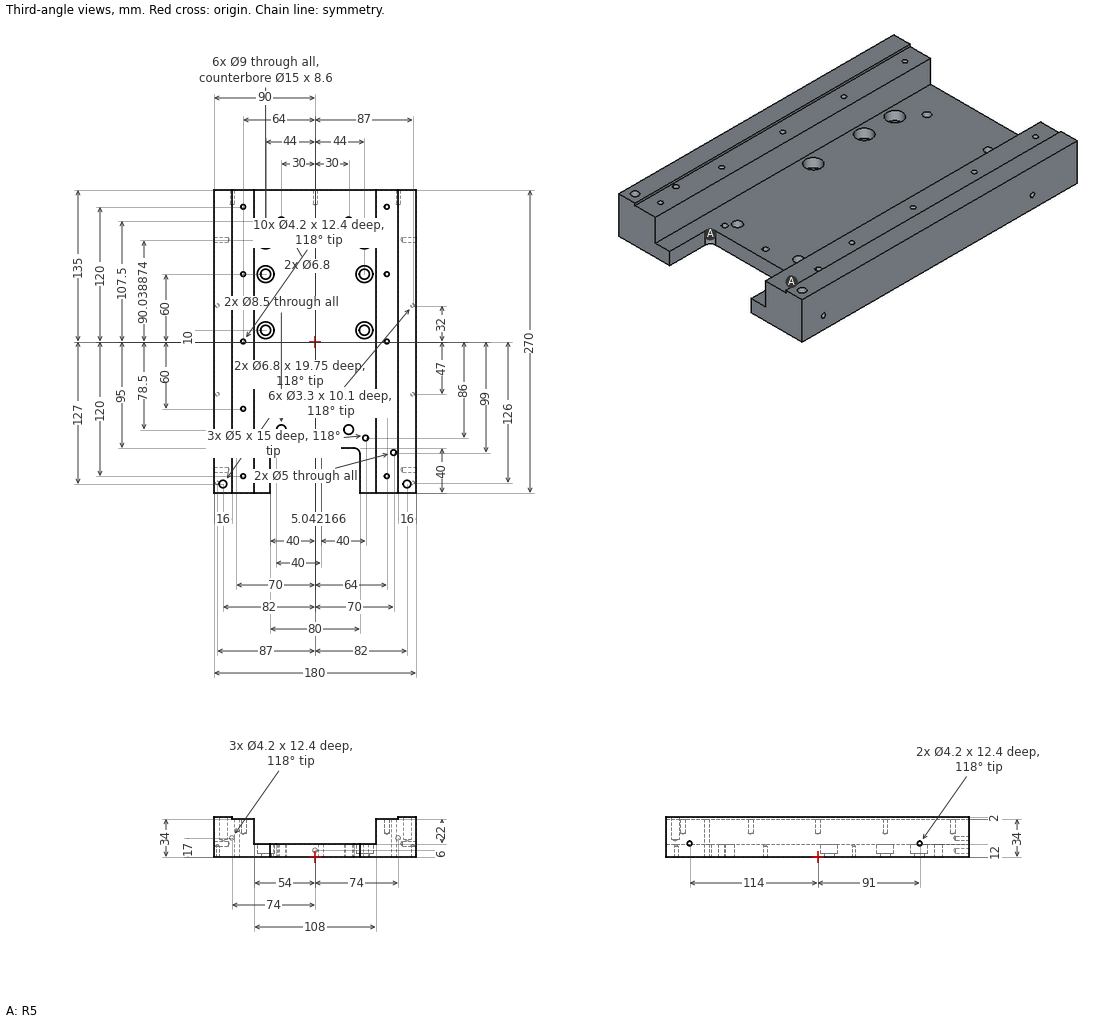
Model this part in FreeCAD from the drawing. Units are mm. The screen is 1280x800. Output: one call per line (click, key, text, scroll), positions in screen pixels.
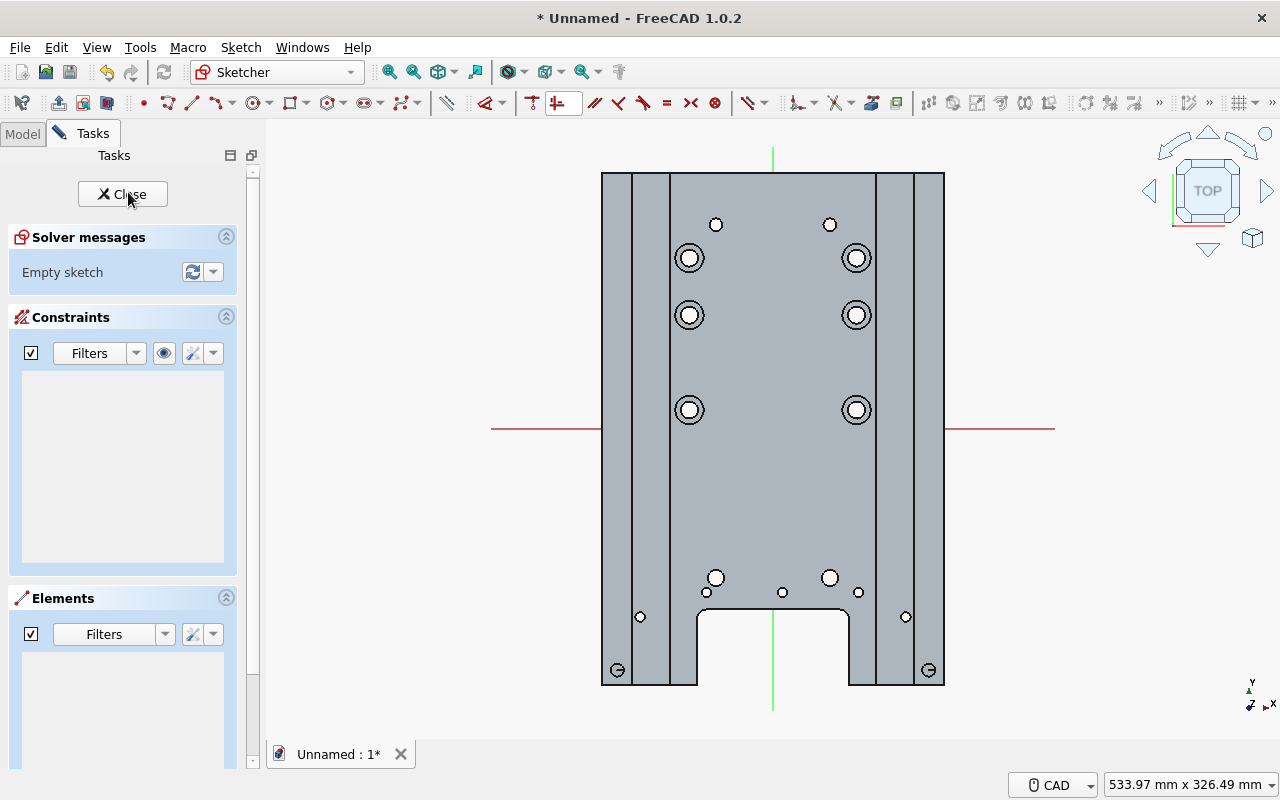
click(108, 104)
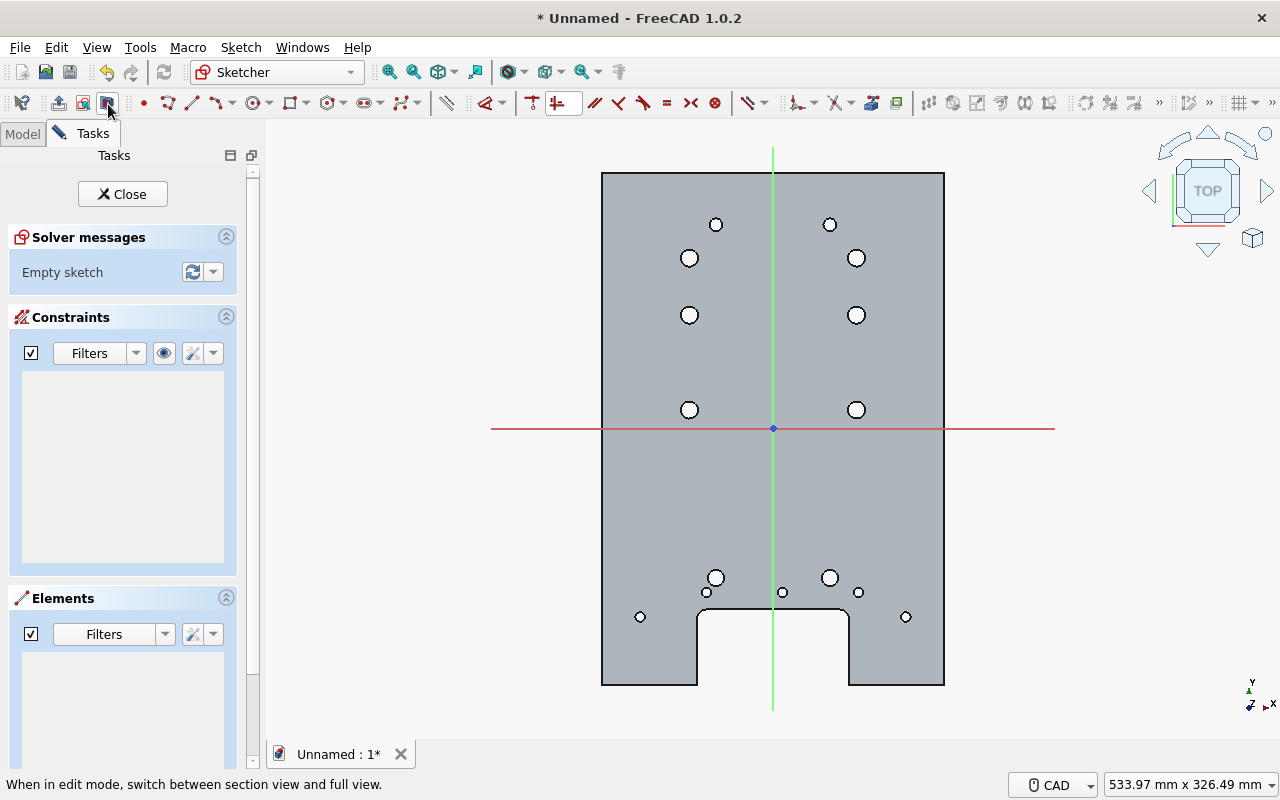
click(254, 104)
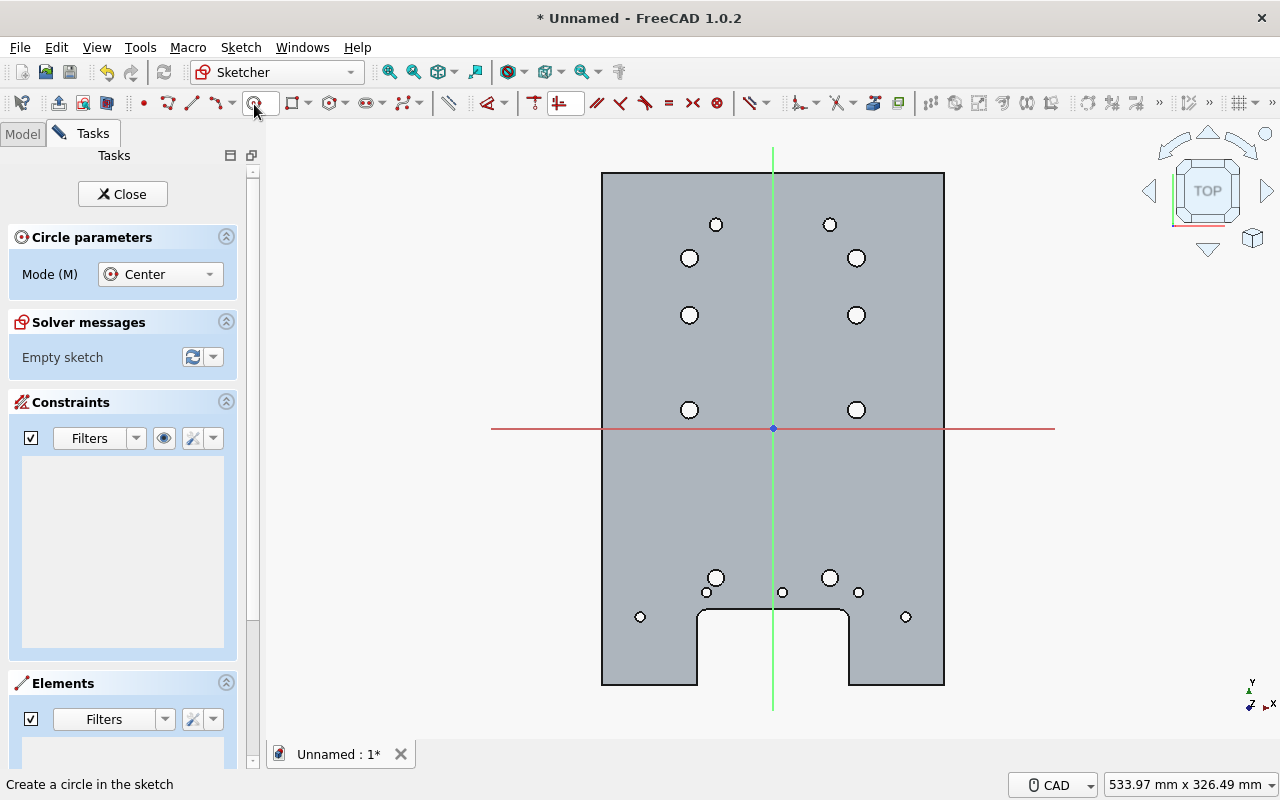
scroll(938, 368, up, 10)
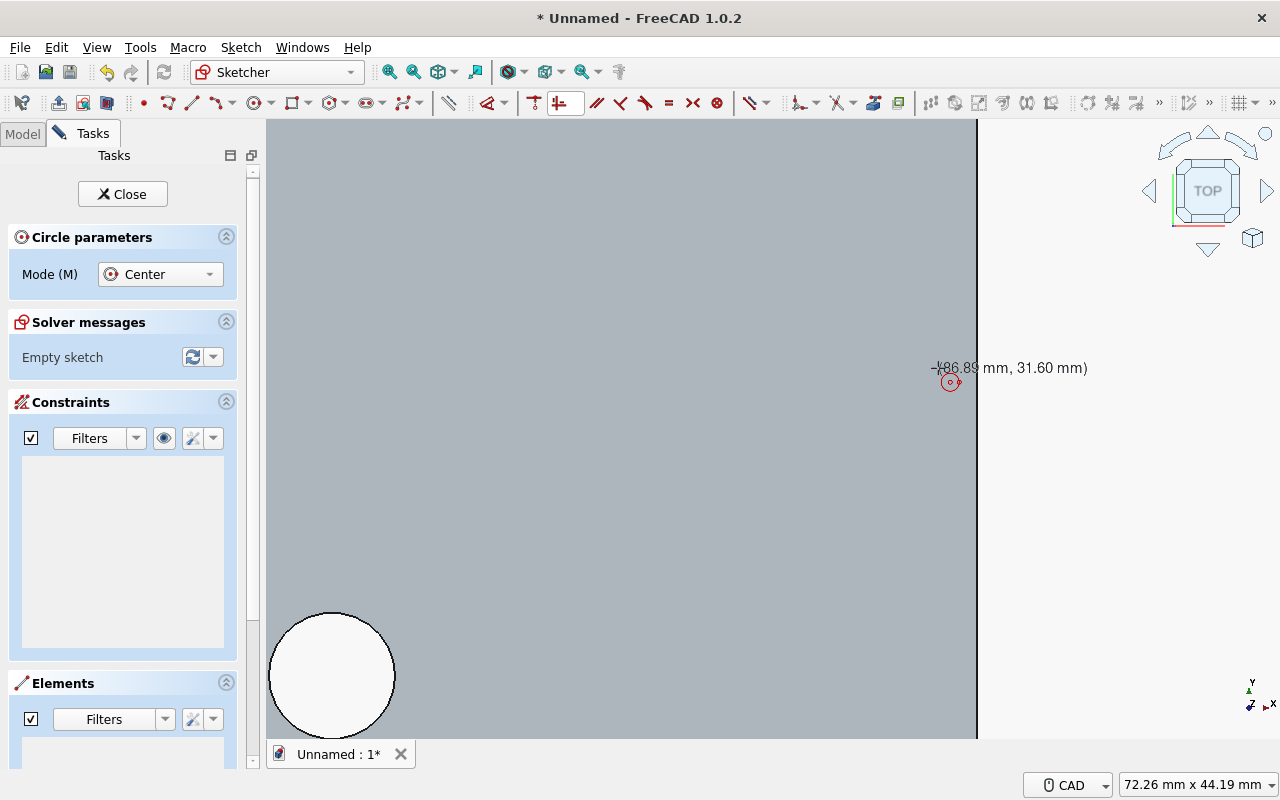
scroll(901, 222, down, 9)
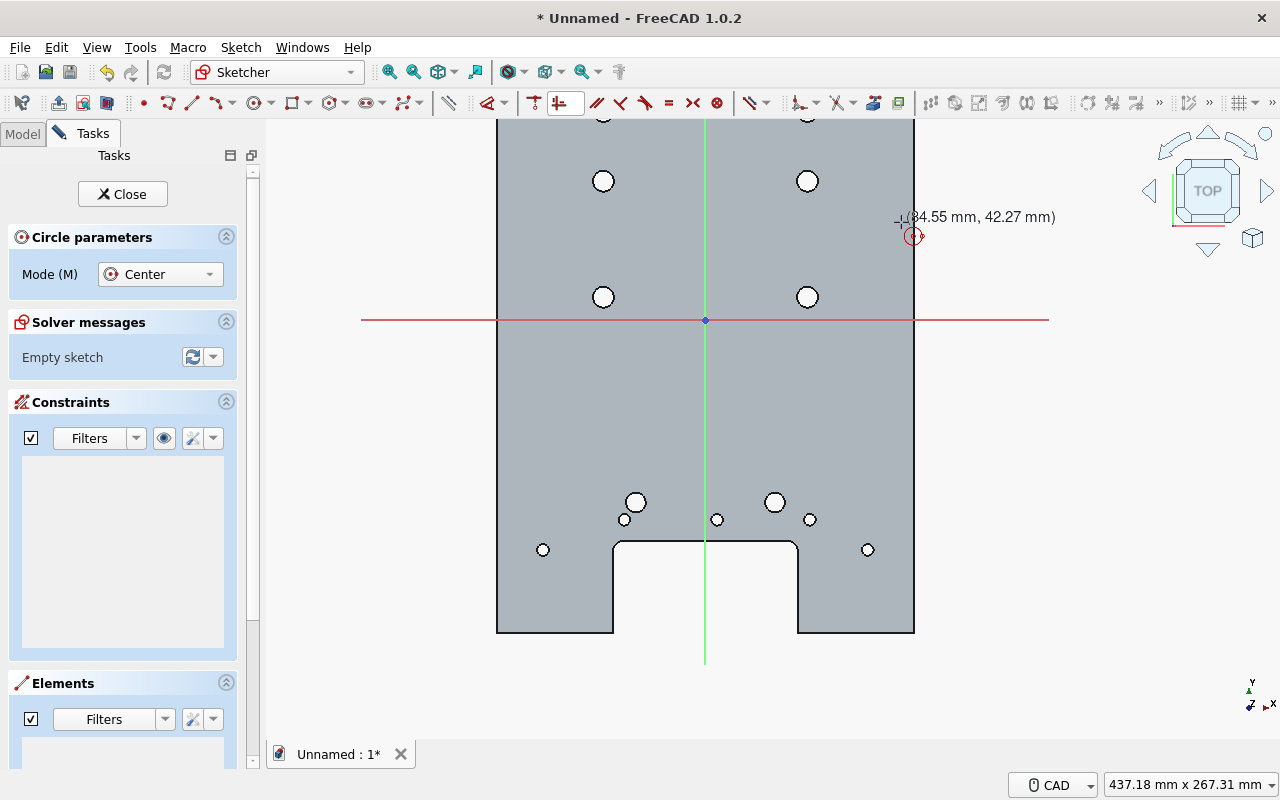
click(907, 246)
move(910, 243)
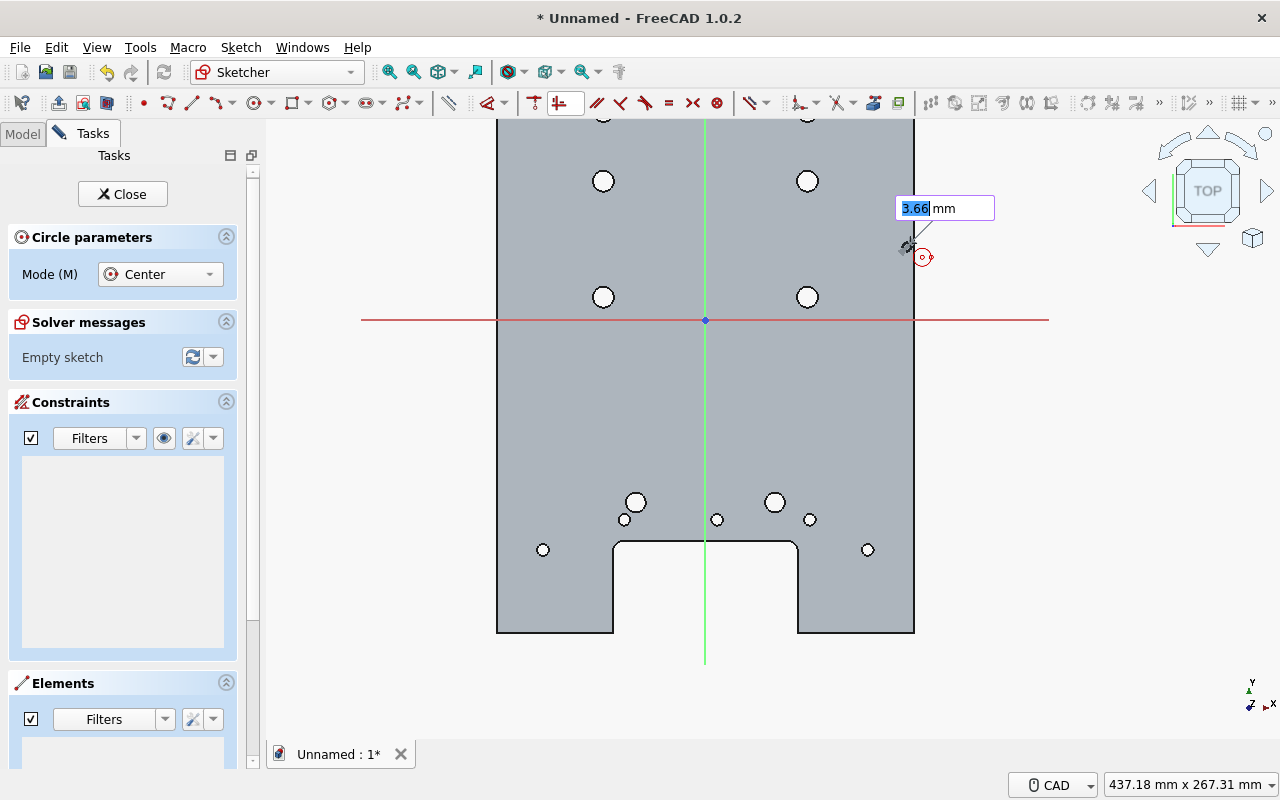
text(3.3)
key(Return)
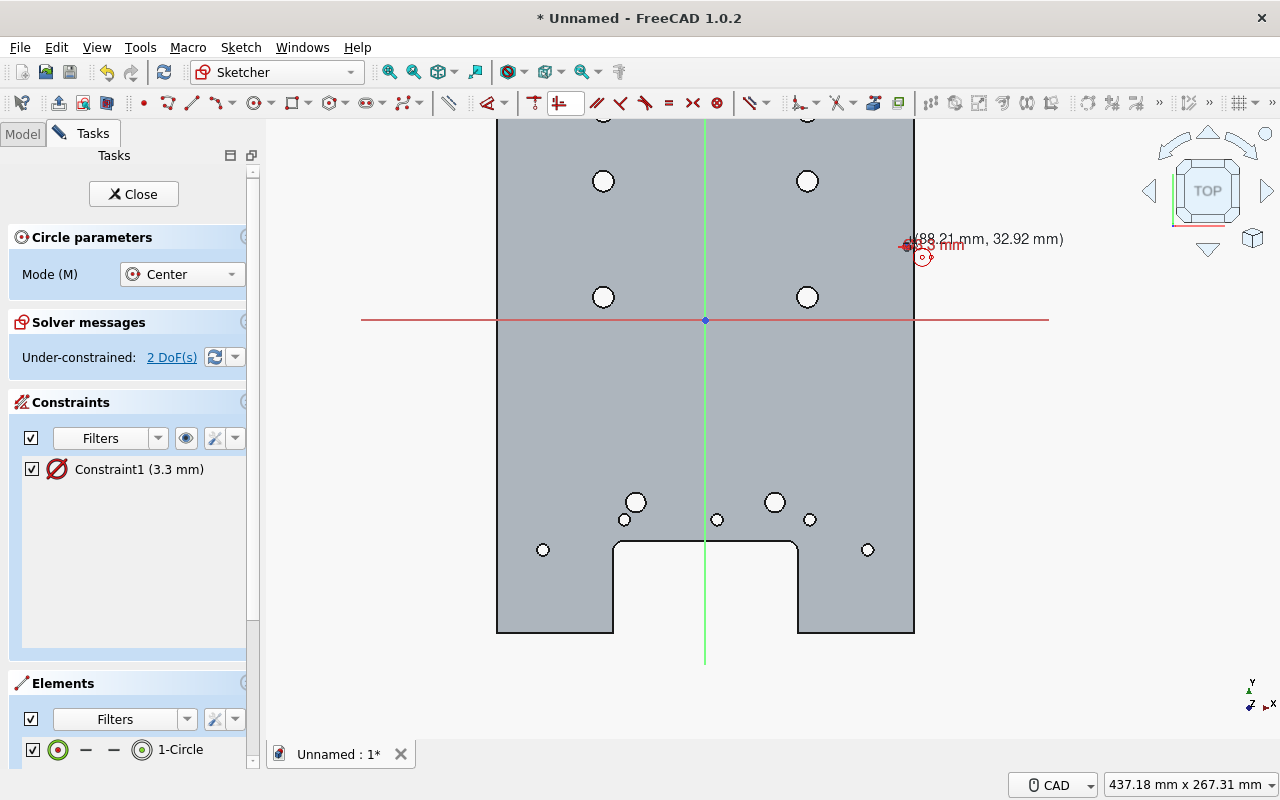
scroll(907, 429, up, 9)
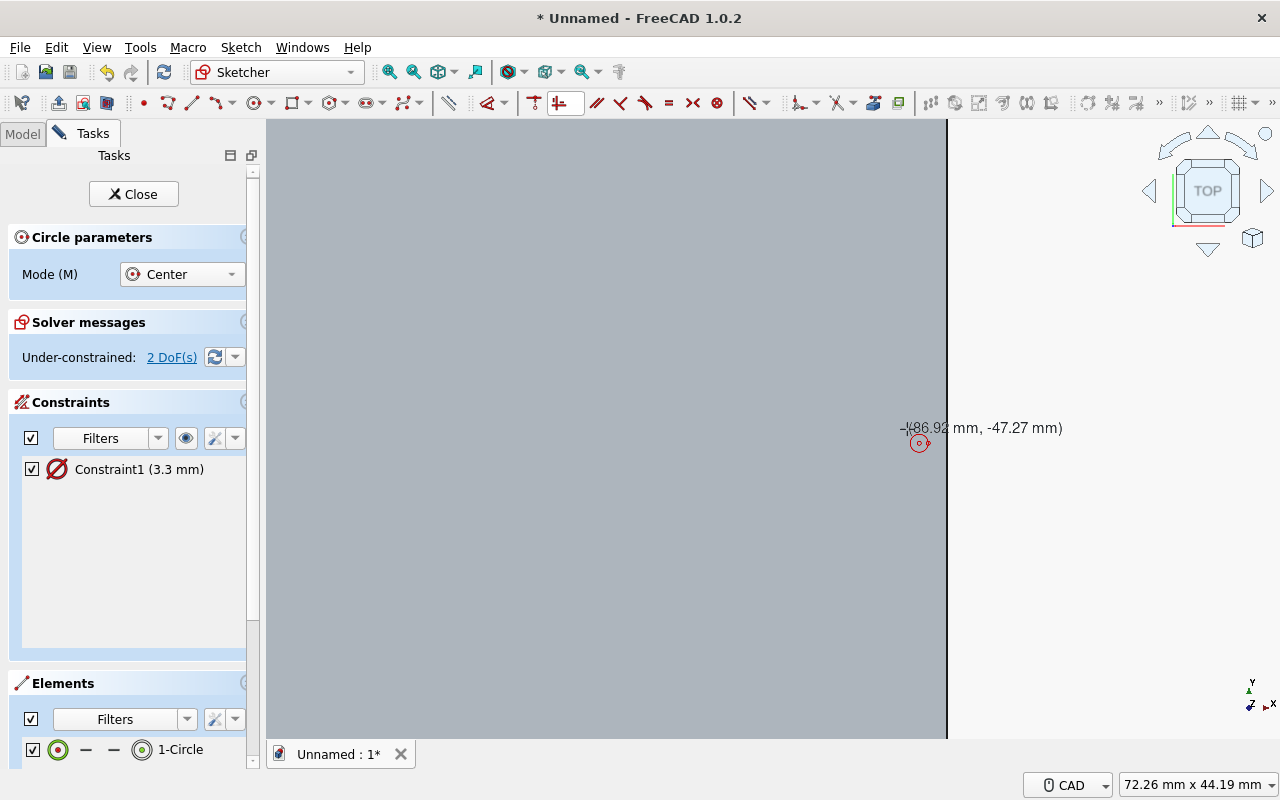
scroll(907, 429, down, 9)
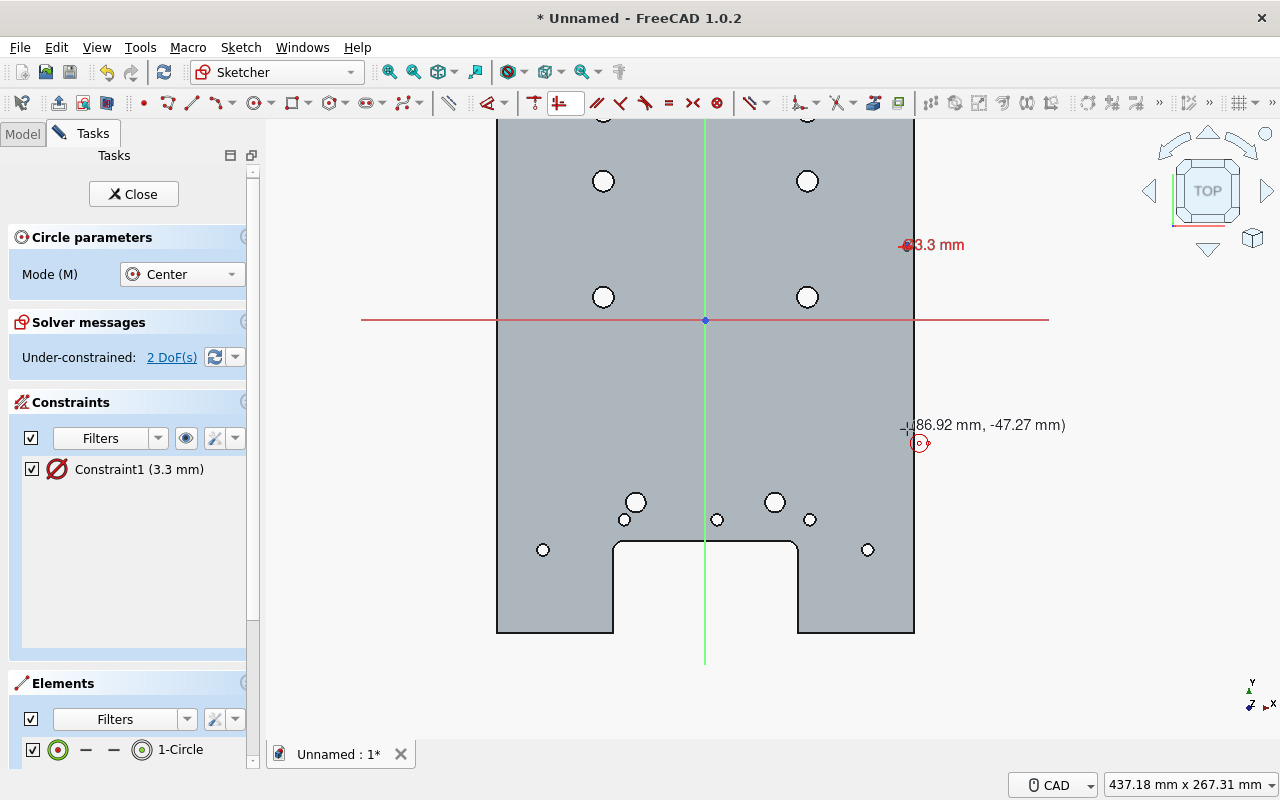
click(907, 429)
move(910, 427)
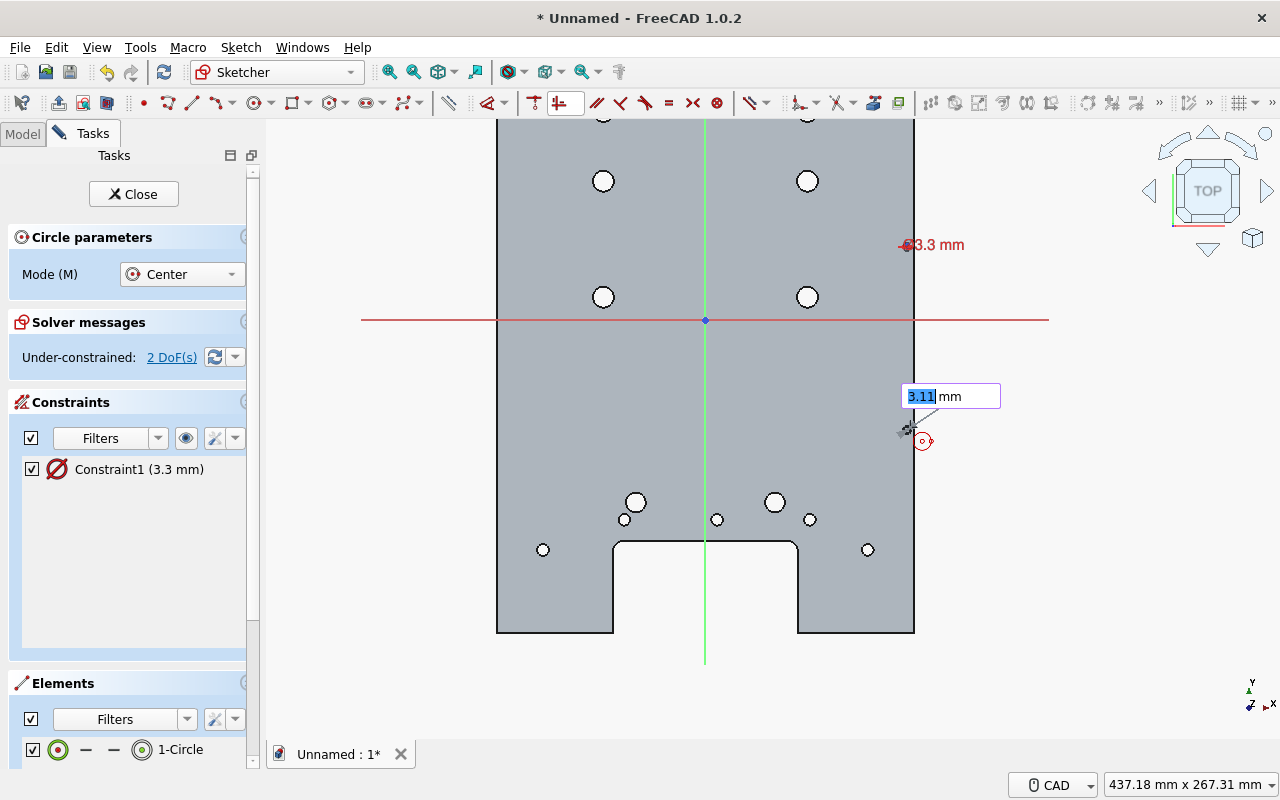
text(3.3)
key(Return)